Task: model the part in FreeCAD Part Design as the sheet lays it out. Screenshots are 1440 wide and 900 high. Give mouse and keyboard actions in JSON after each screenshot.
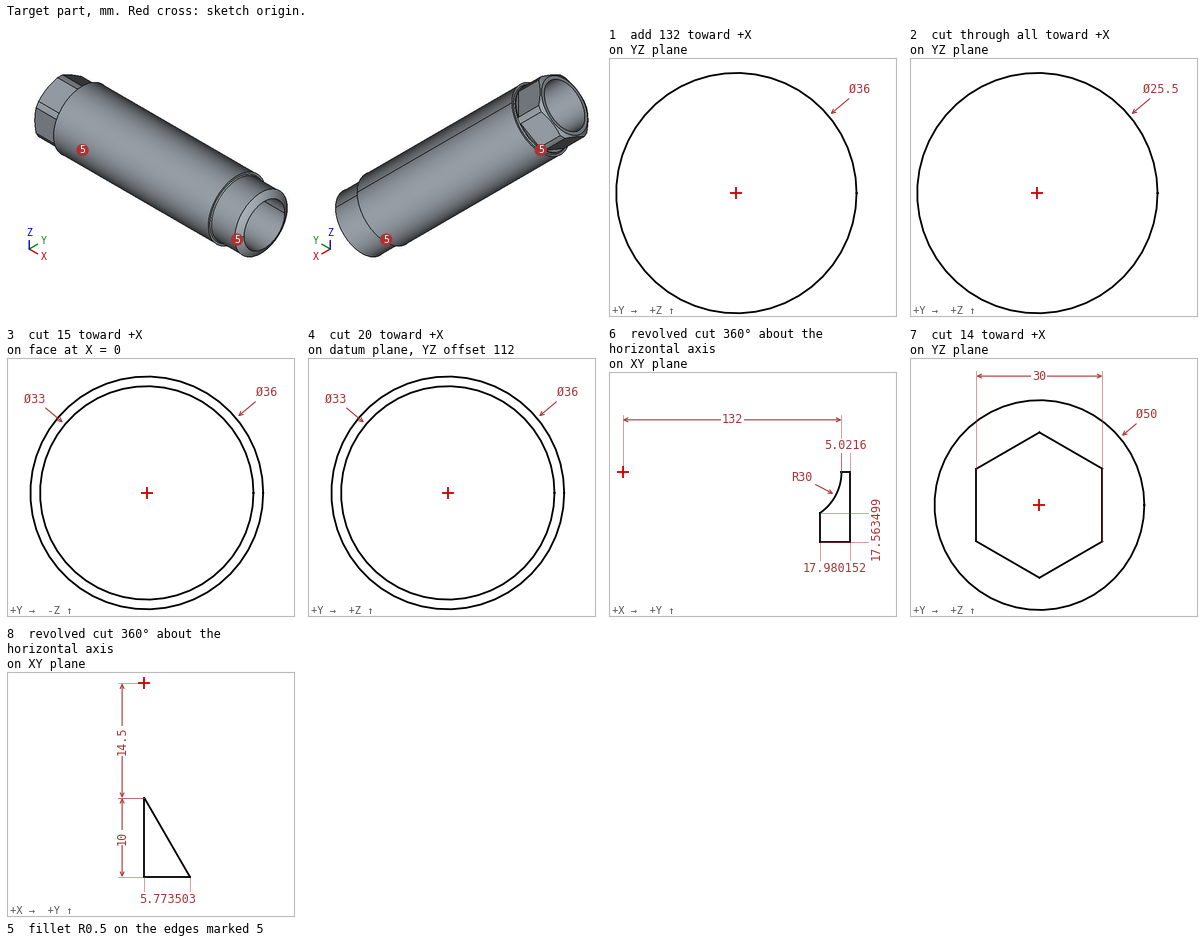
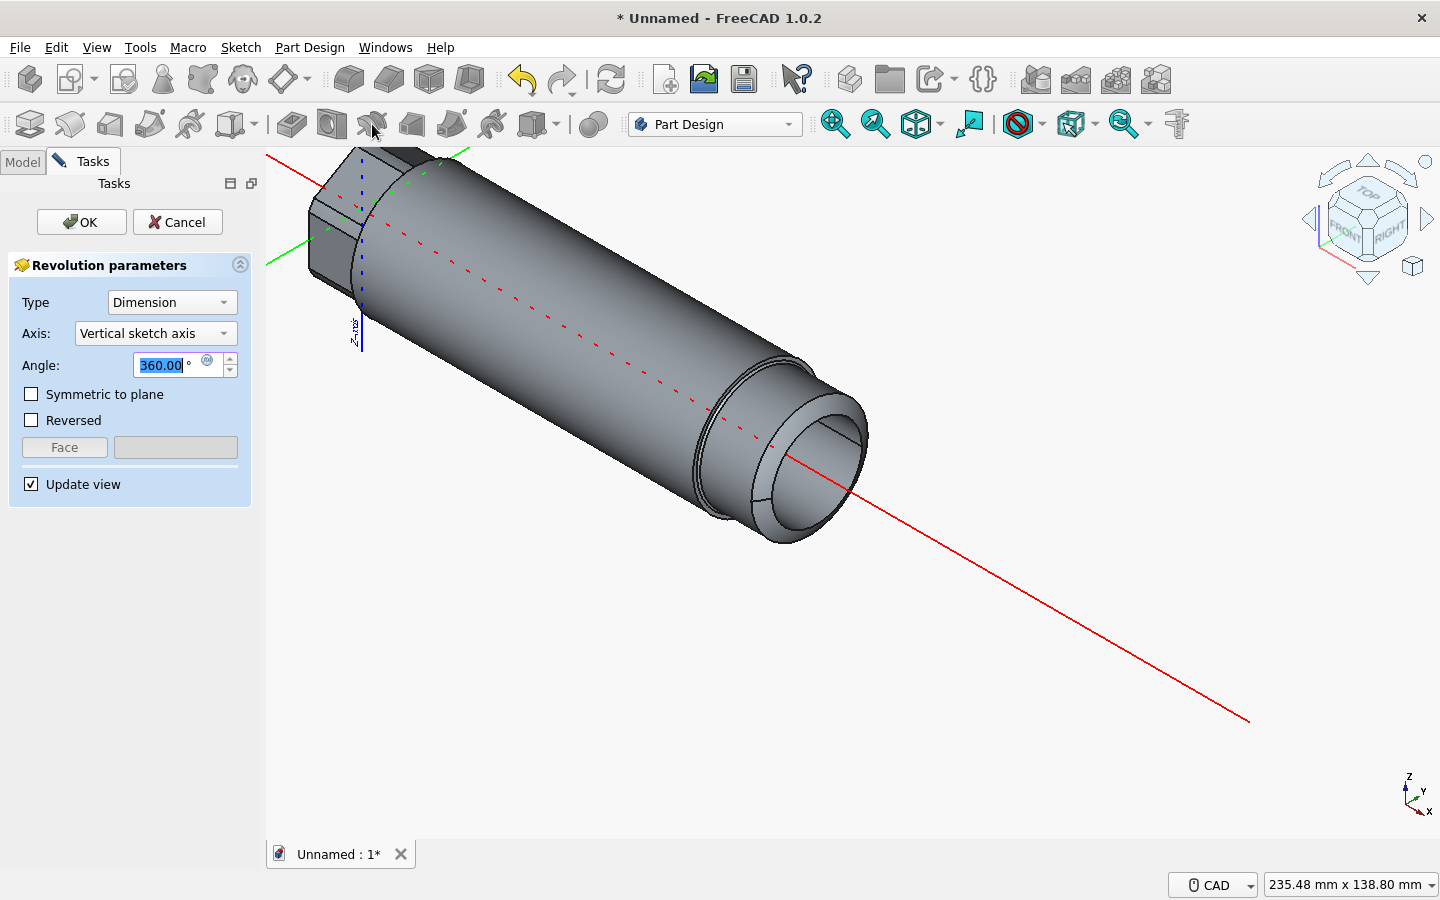
{"action": "left_click", "coordinate": [156, 334]}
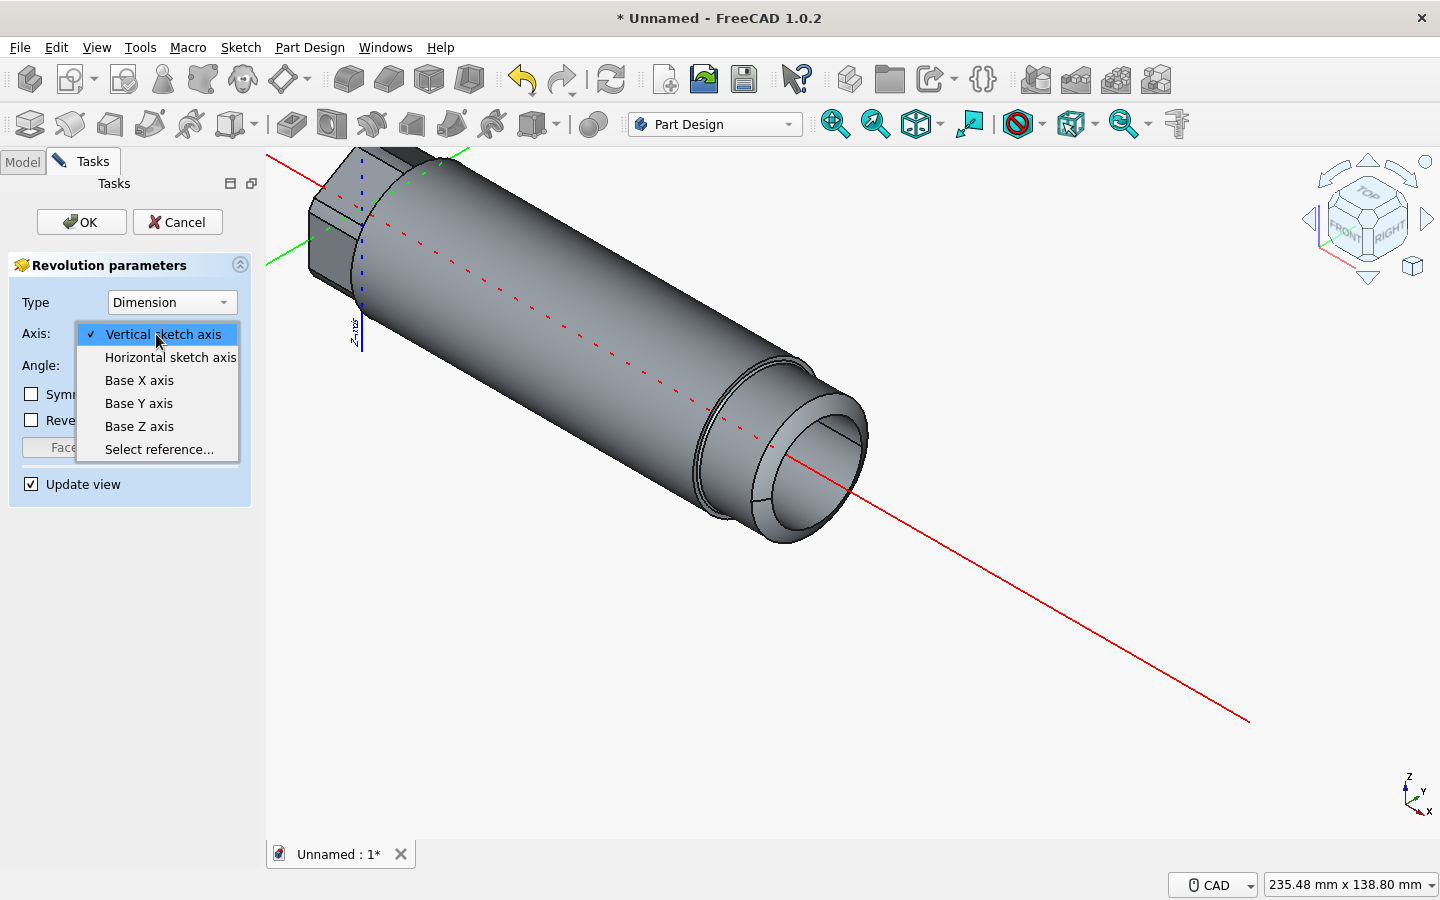
{"action": "left_click", "coordinate": [156, 358]}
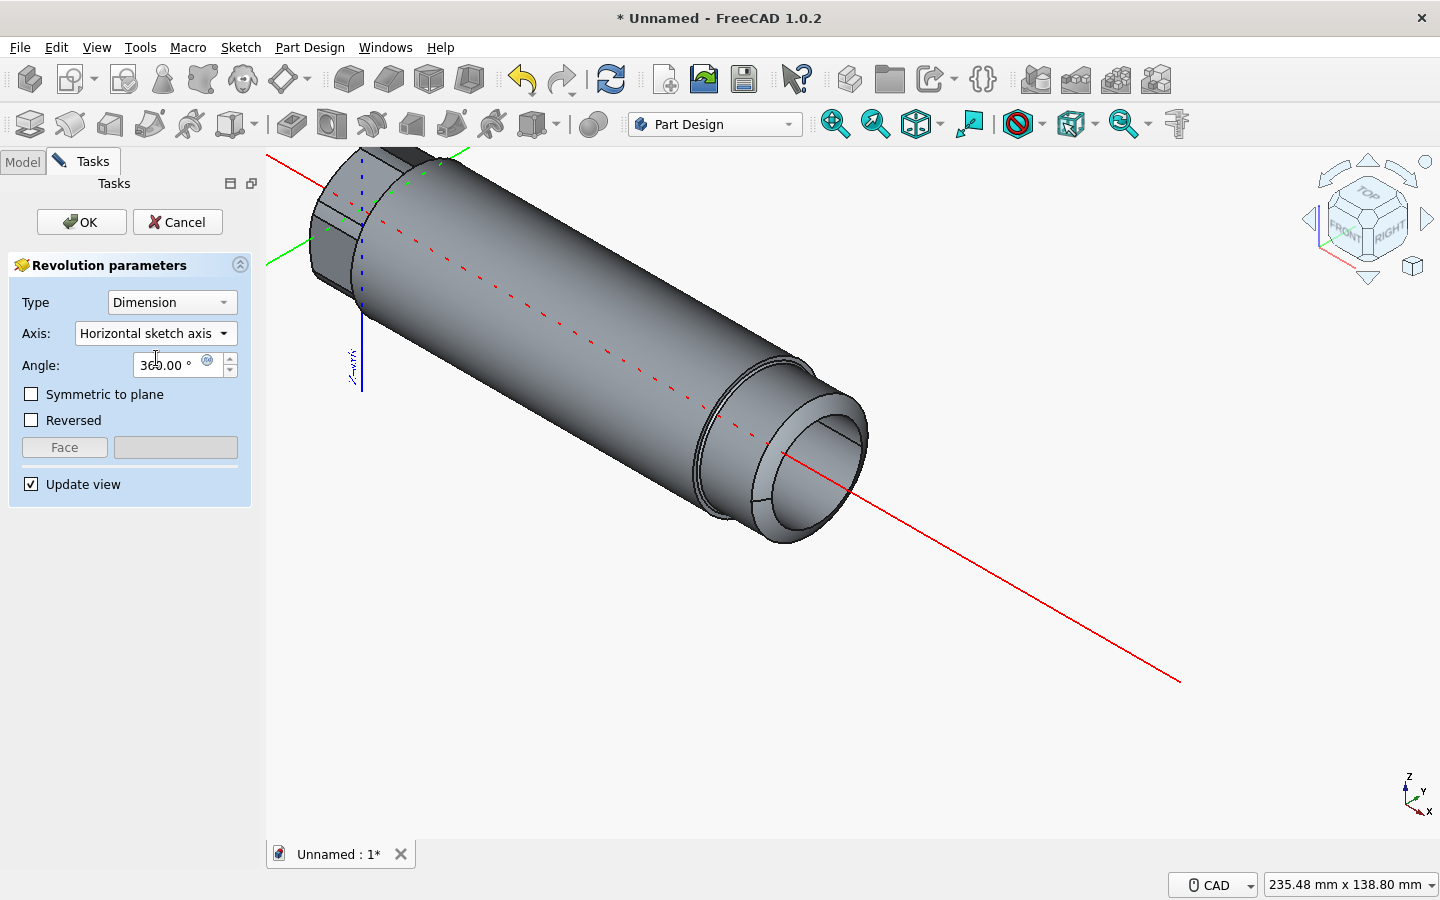
{"action": "left_click", "coordinate": [82, 222]}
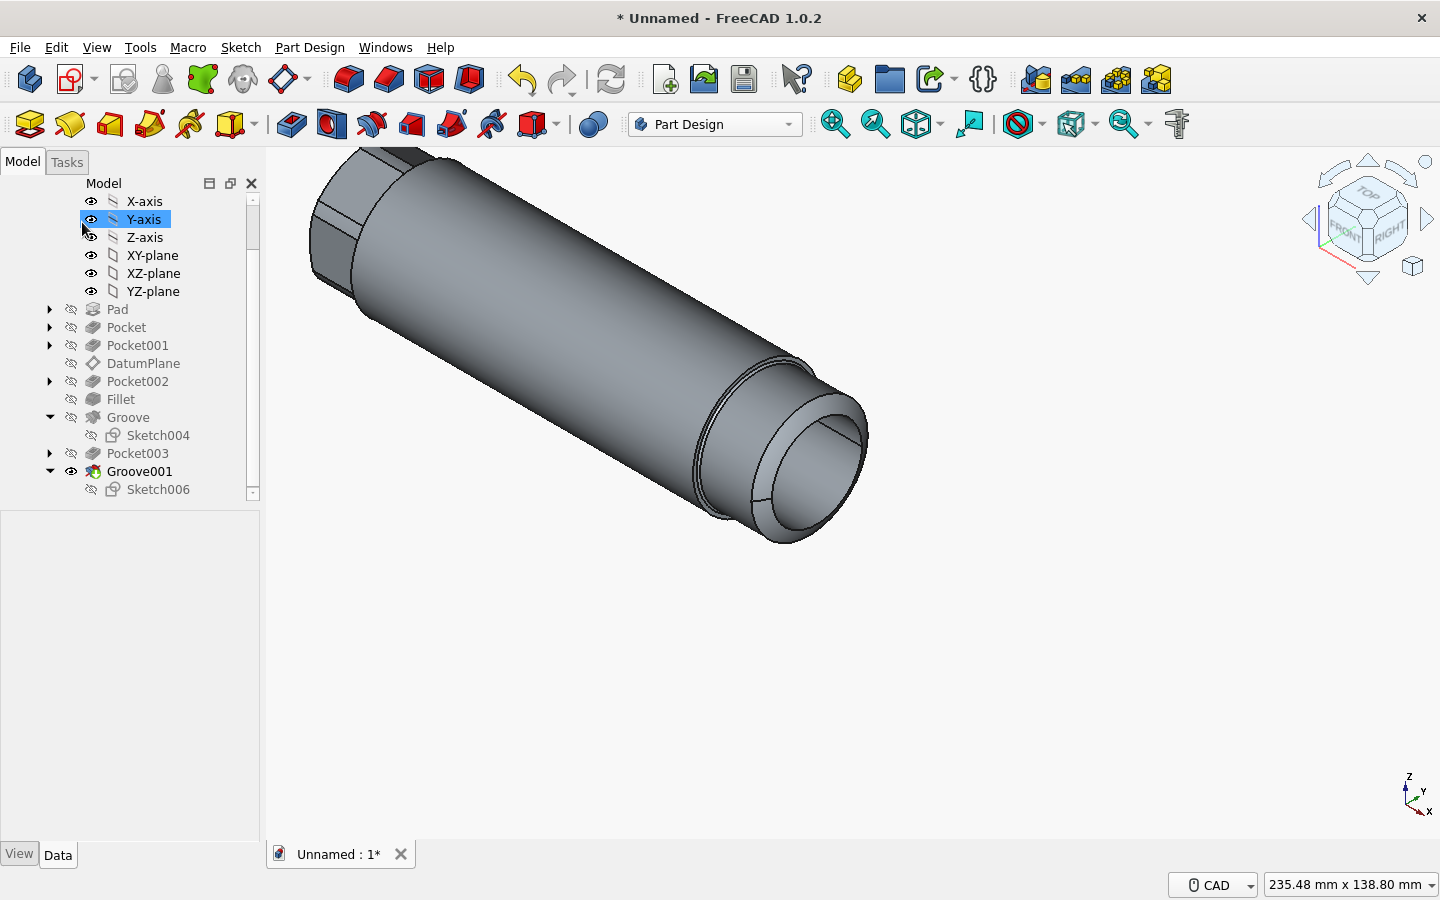
{"action": "left_click", "coordinate": [836, 124]}